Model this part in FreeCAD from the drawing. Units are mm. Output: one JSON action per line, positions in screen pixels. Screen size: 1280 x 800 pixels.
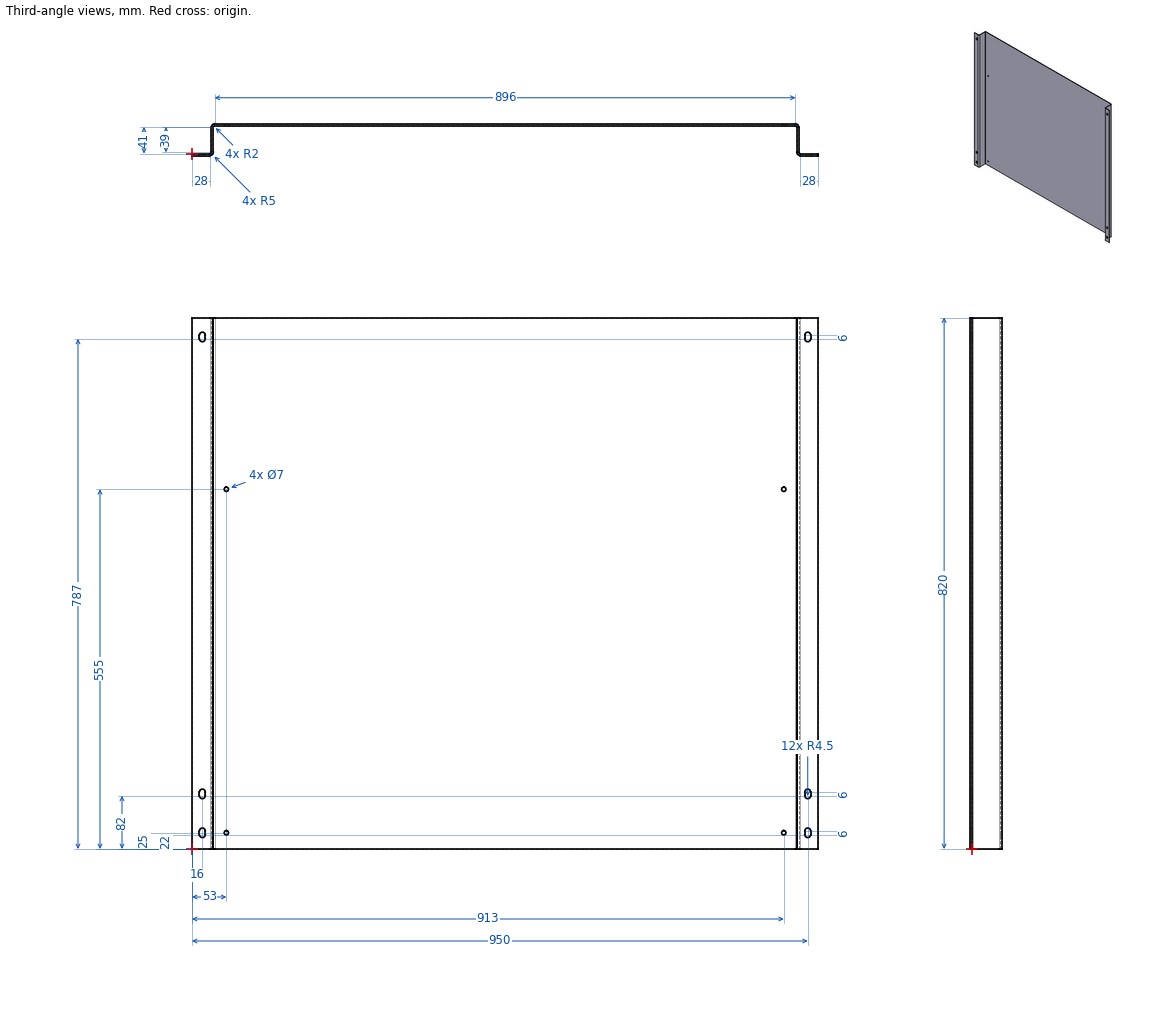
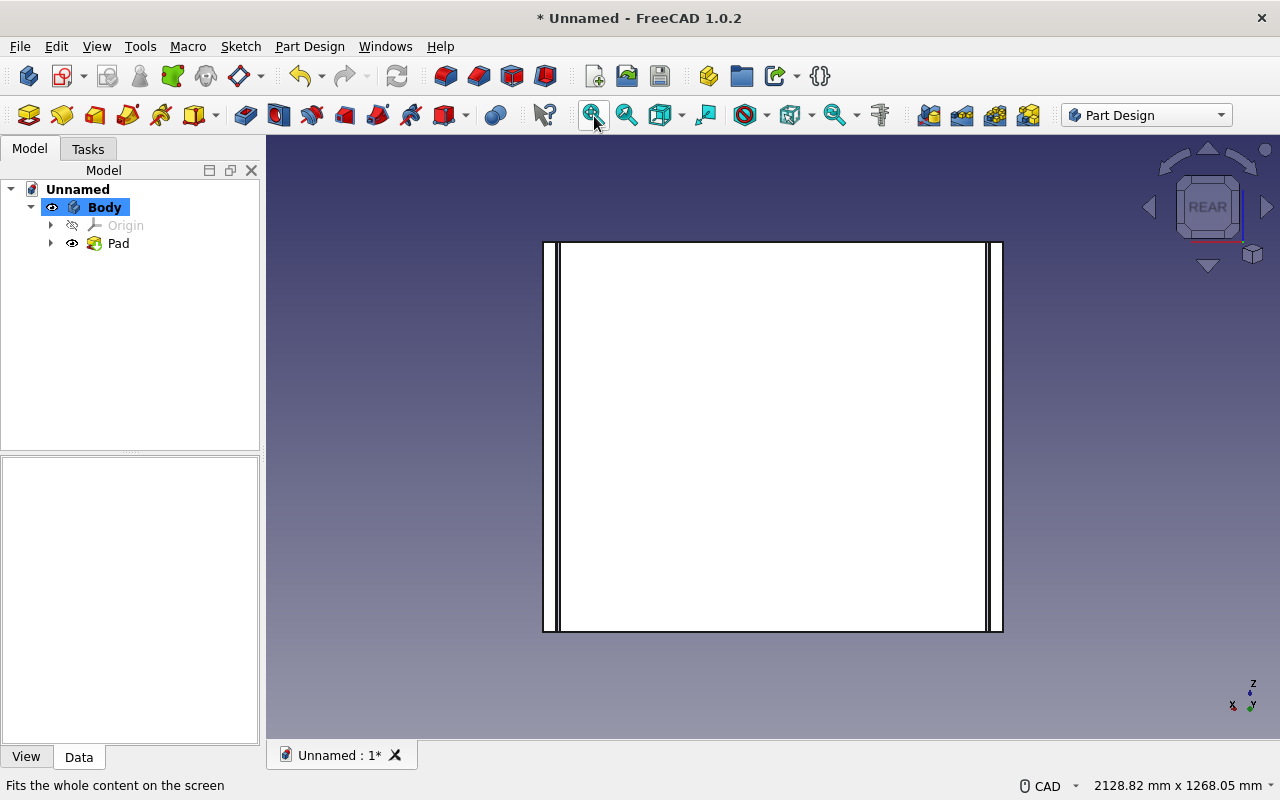
{"action": "left_click", "coordinate": [773, 436]}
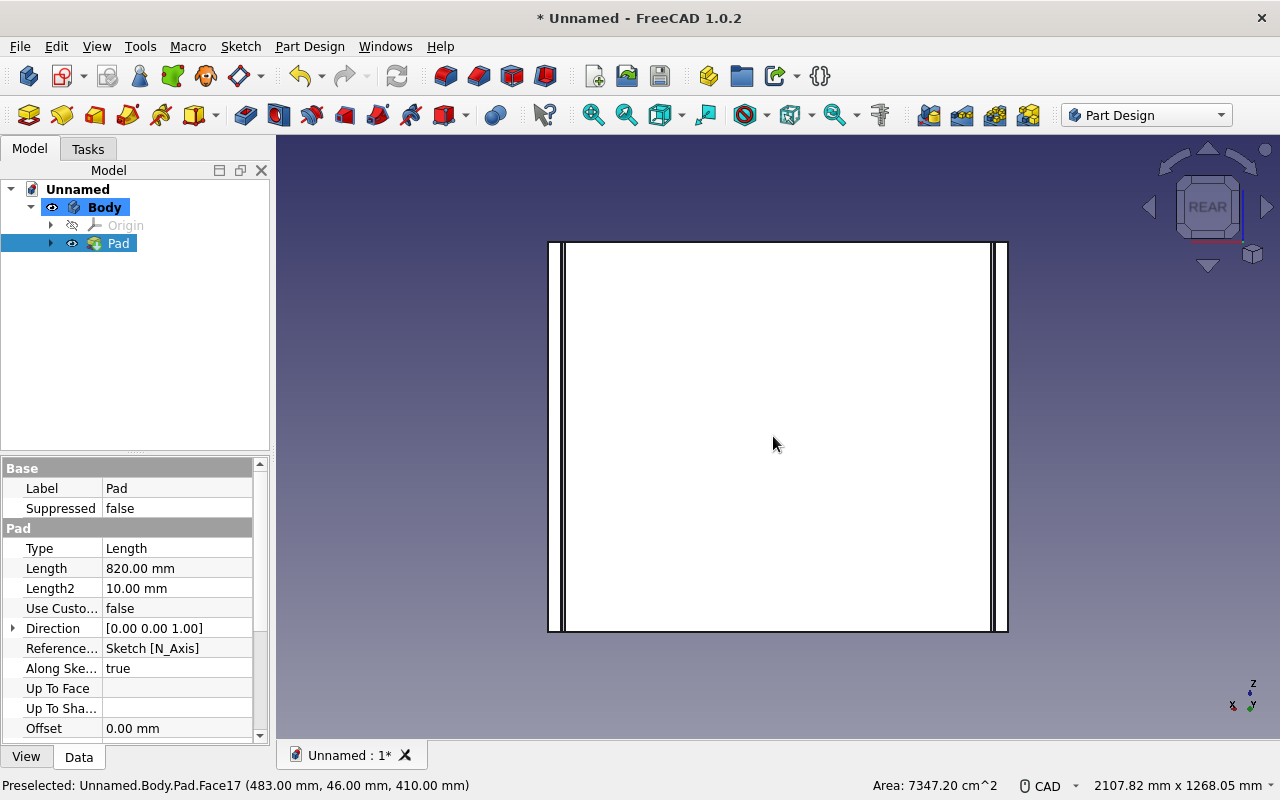
{"action": "left_click", "coordinate": [62, 76]}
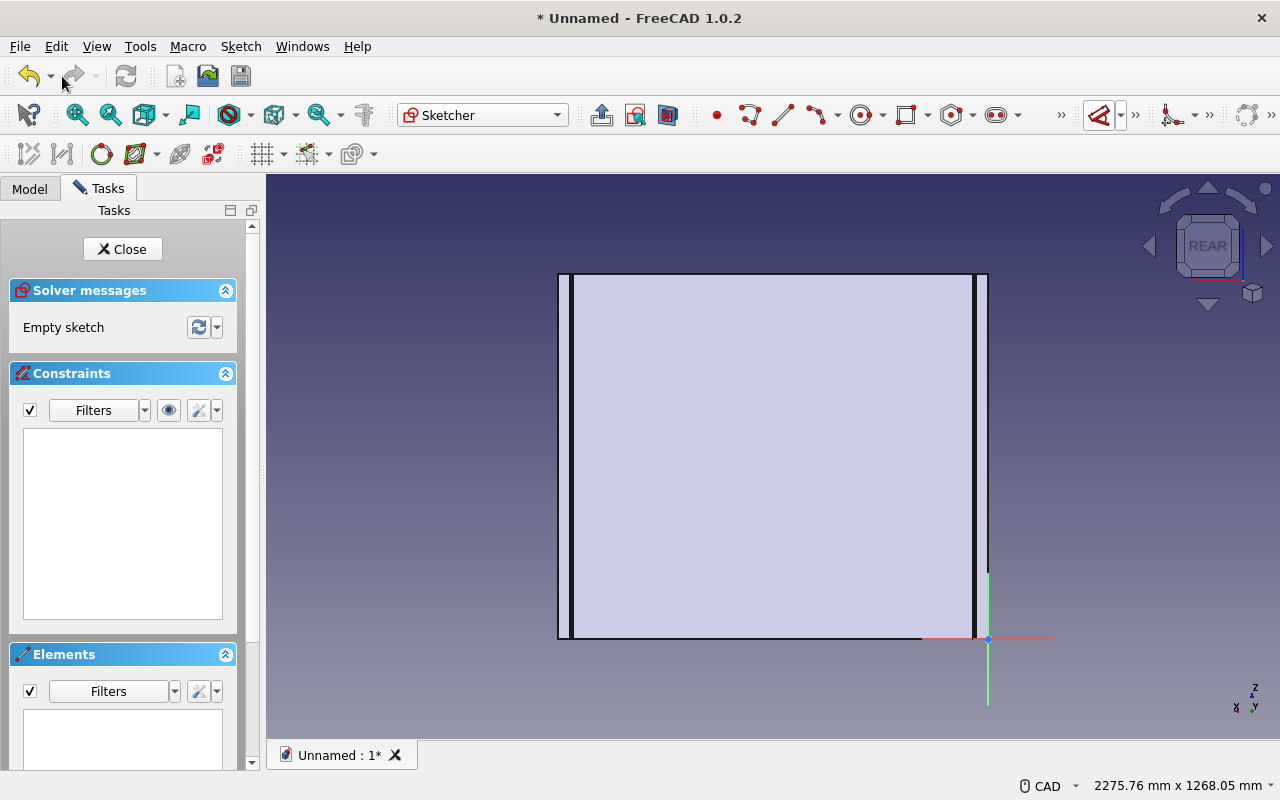
{"action": "scroll", "coordinate": [946, 633], "scroll_direction": "up", "scroll_amount": 2}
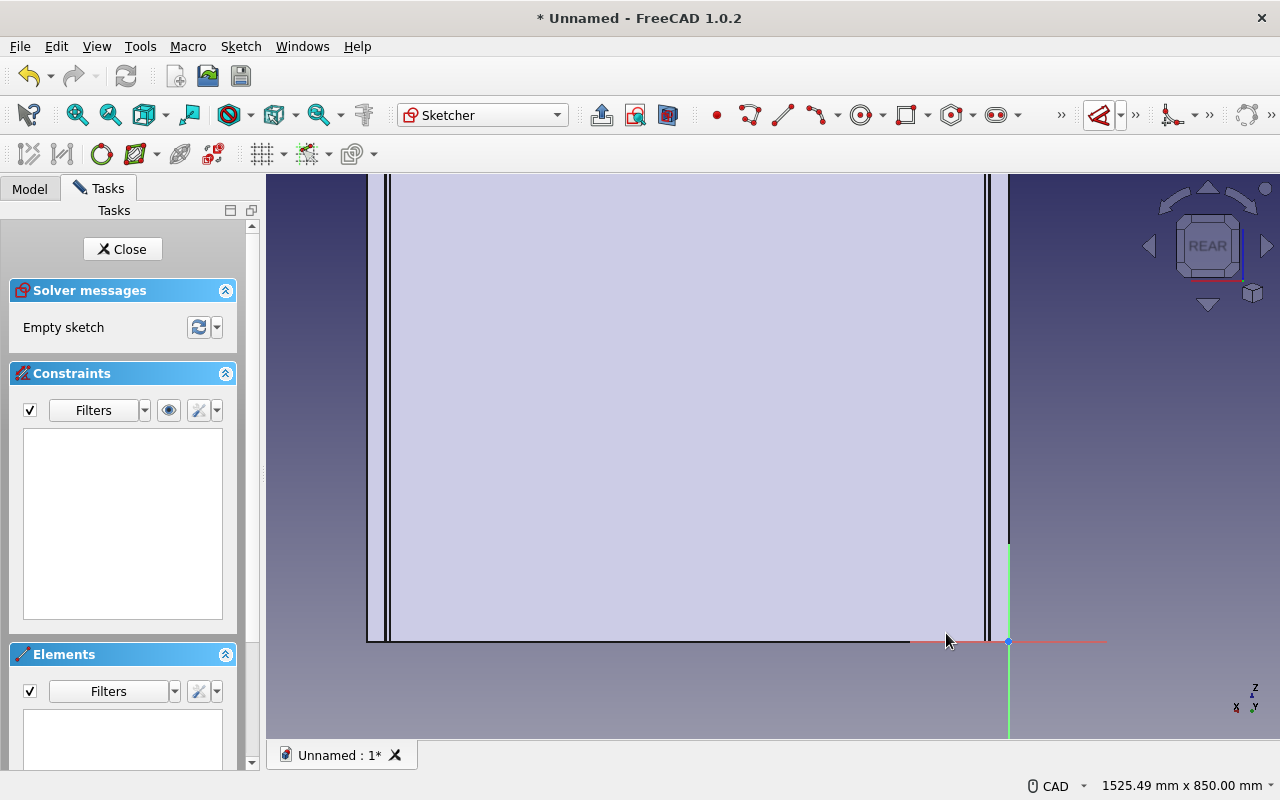
{"action": "left_click", "coordinate": [860, 116]}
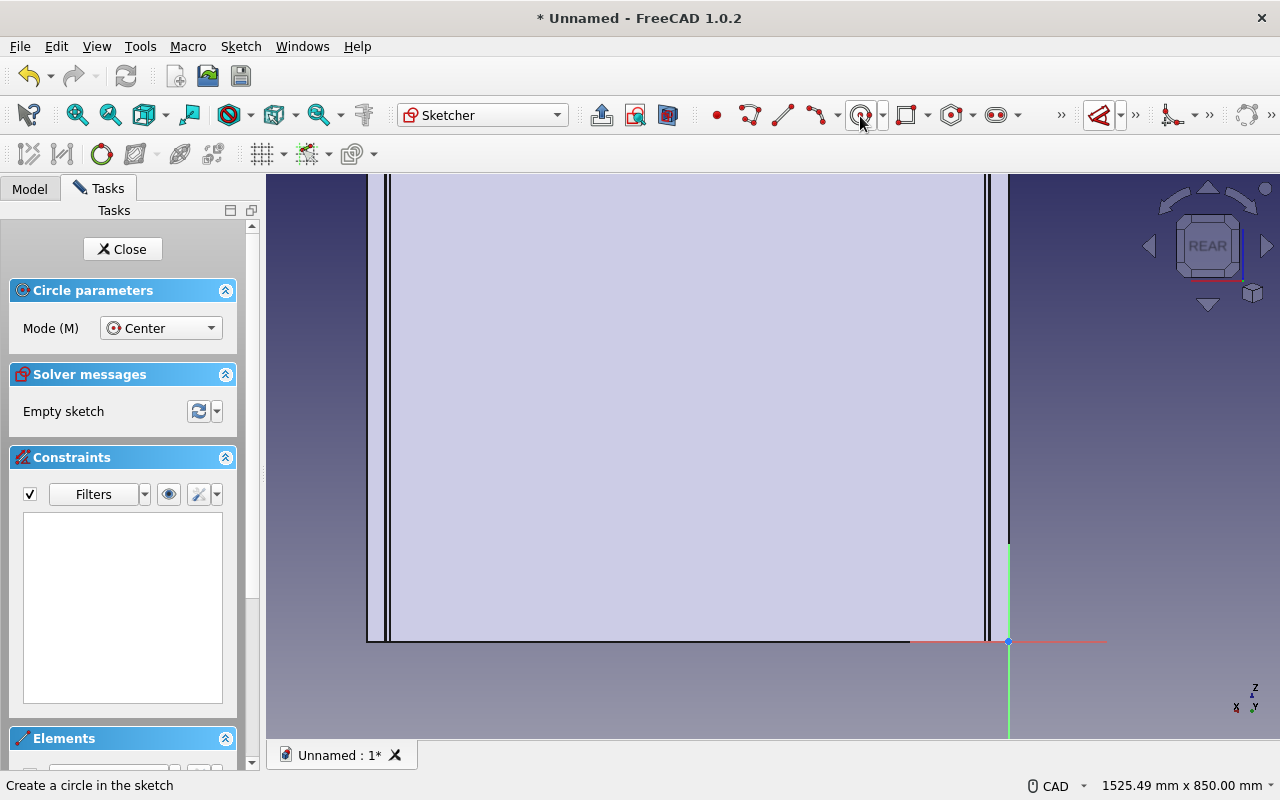
{"action": "scroll", "coordinate": [973, 273], "scroll_direction": "up", "scroll_amount": 12}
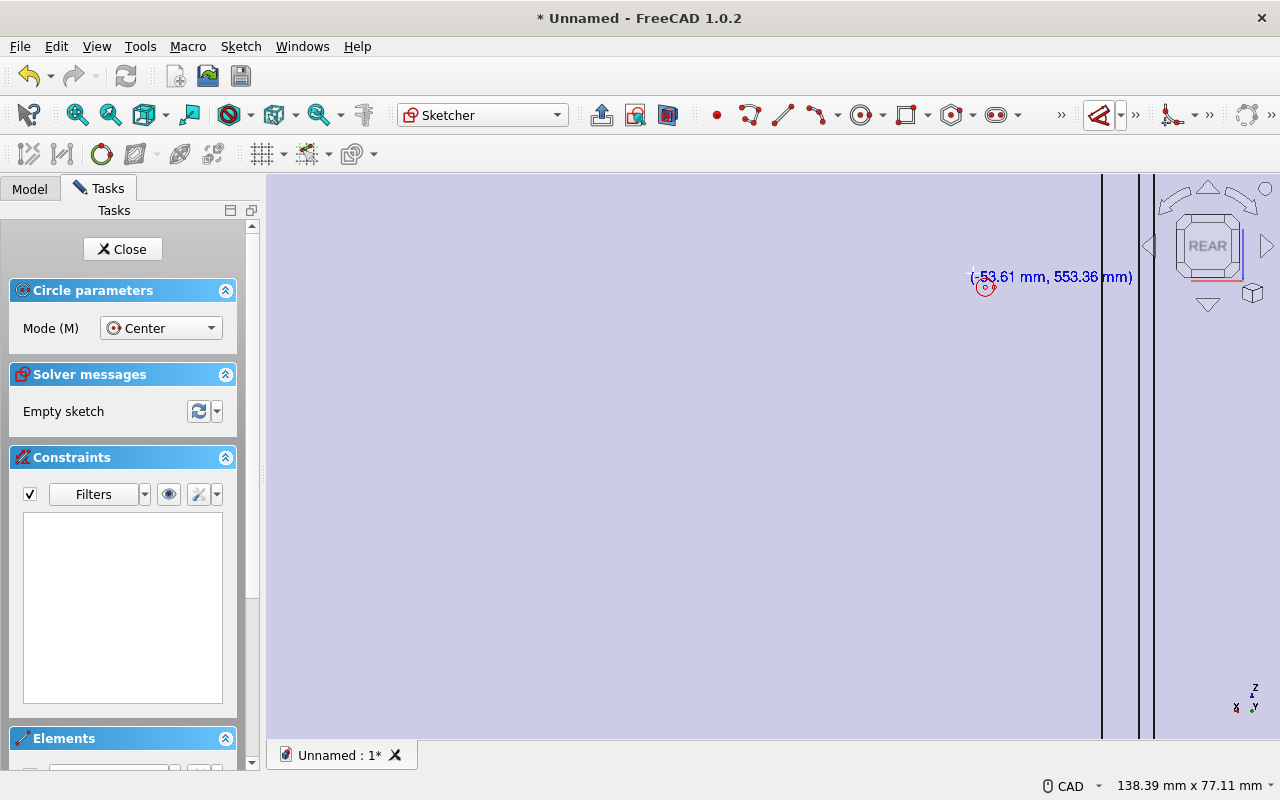
{"action": "scroll", "coordinate": [974, 274], "scroll_direction": "down", "scroll_amount": 12}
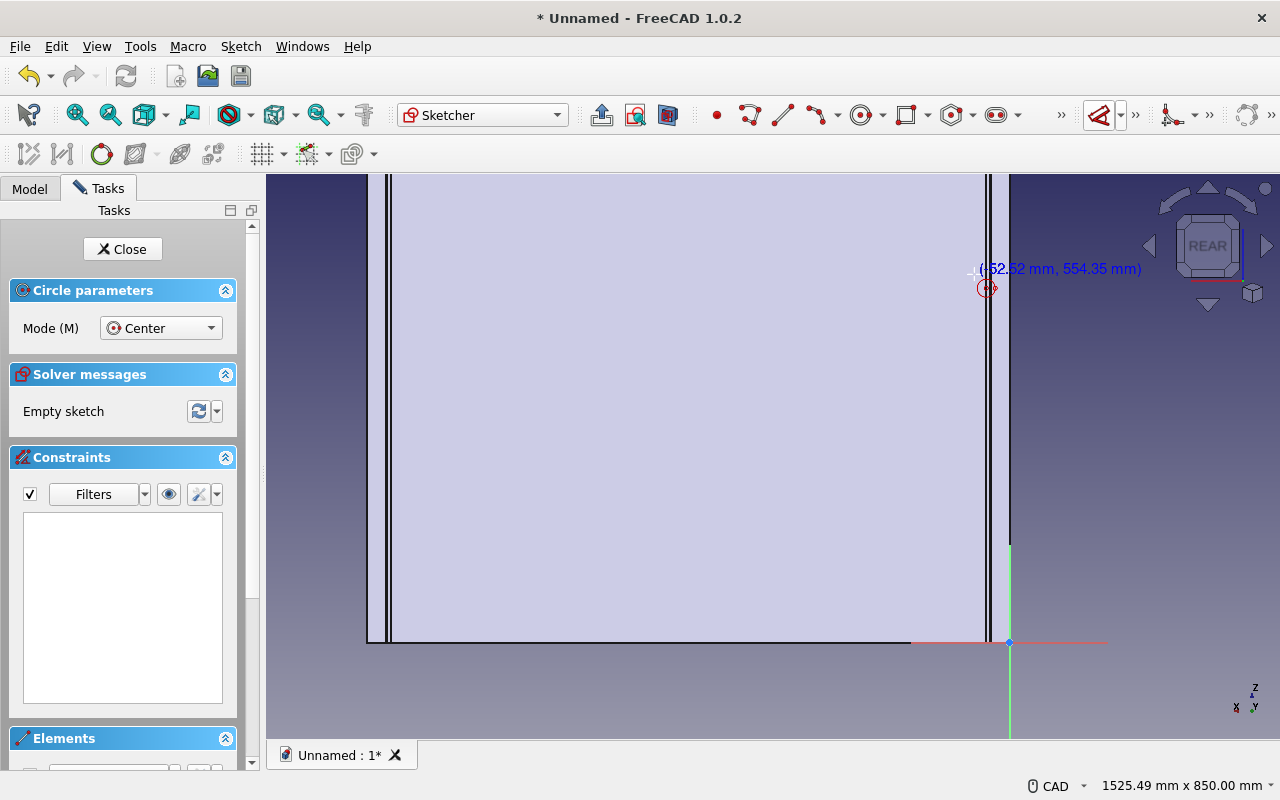
{"action": "left_click", "coordinate": [974, 274]}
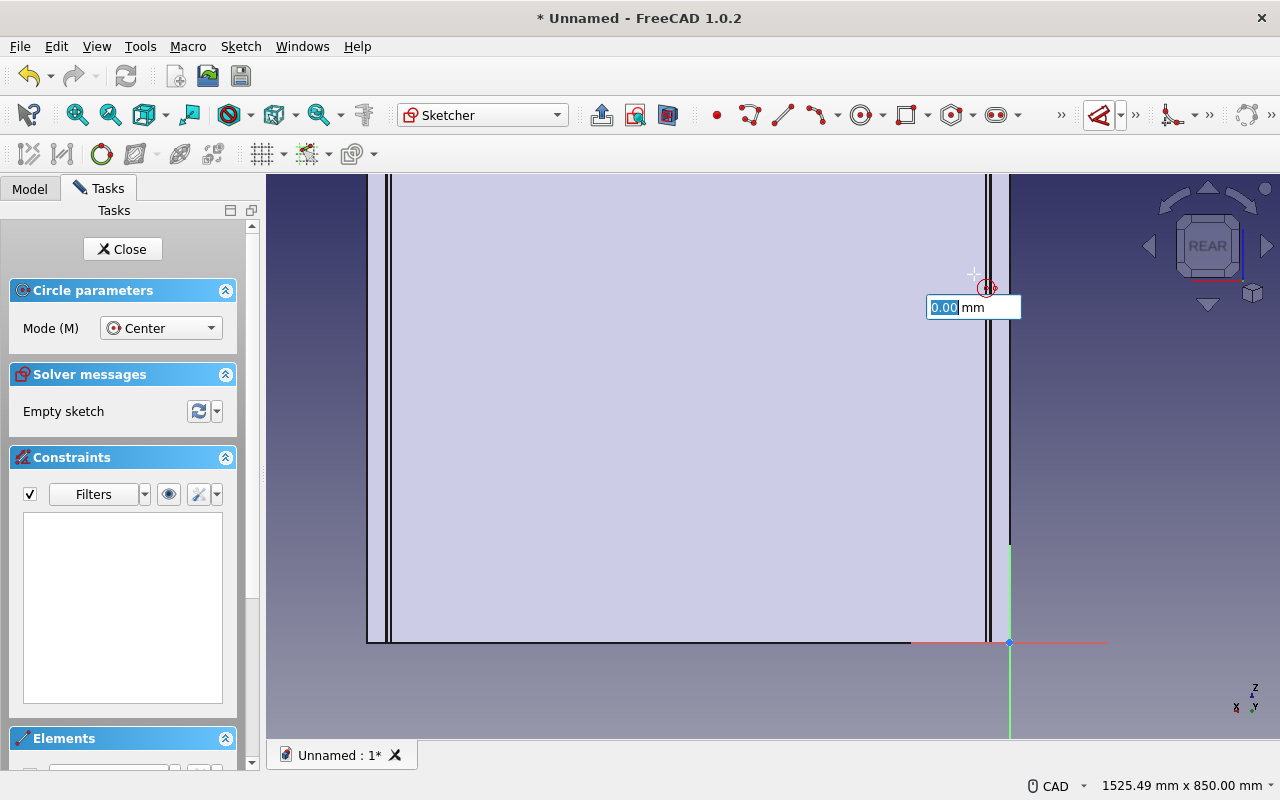
{"action": "scroll", "coordinate": [976, 272], "scroll_direction": "up", "scroll_amount": 10}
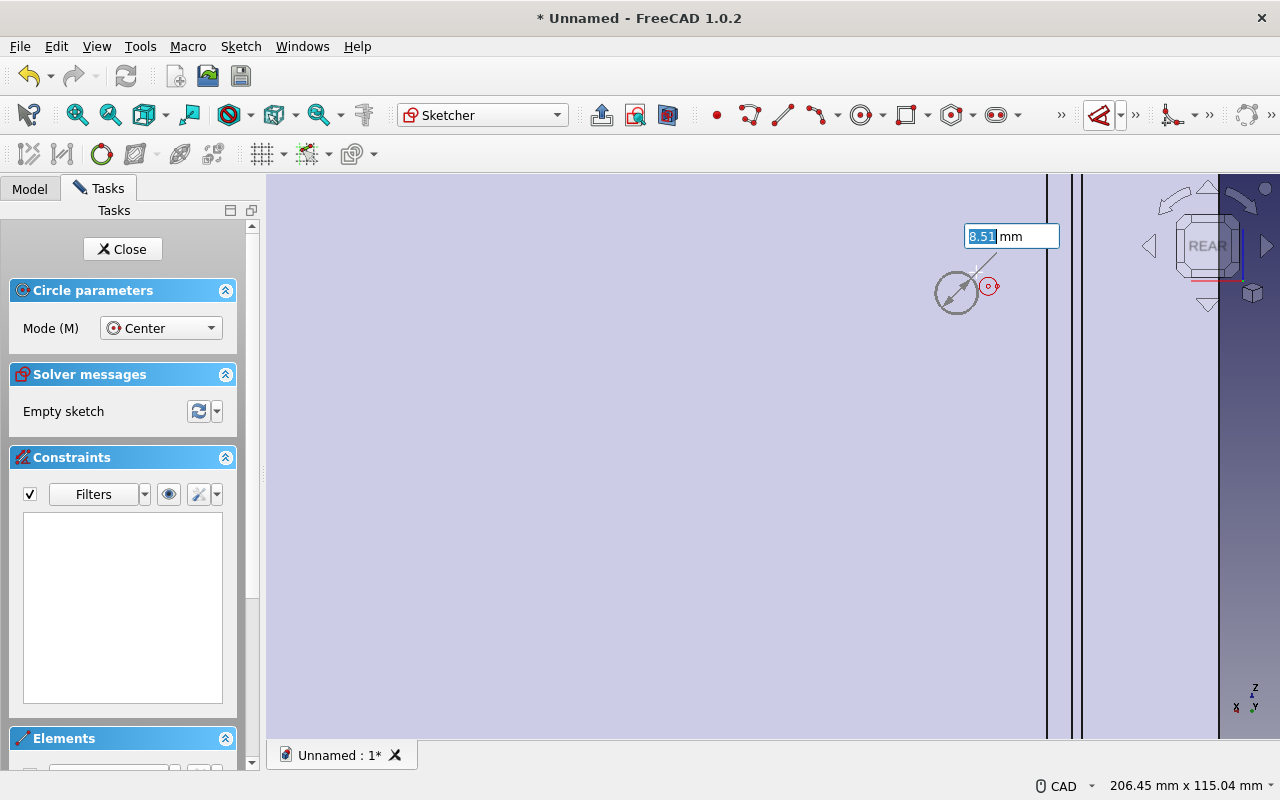
{"action": "left_click", "coordinate": [971, 272]}